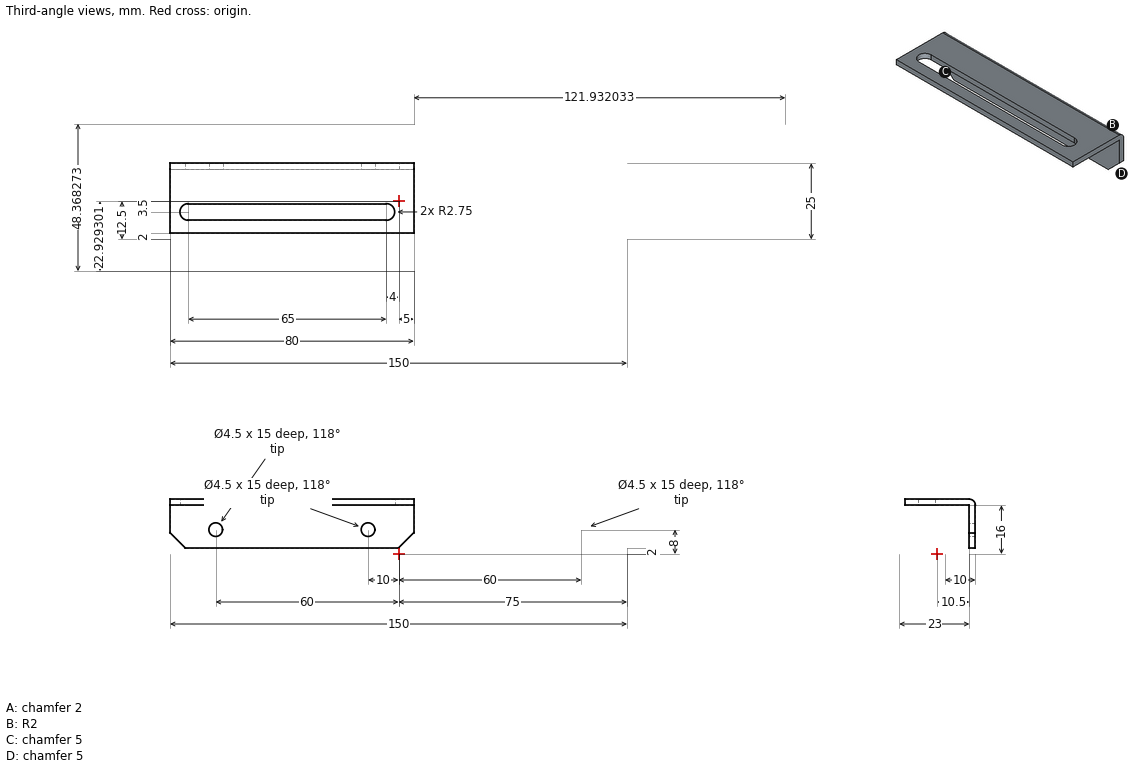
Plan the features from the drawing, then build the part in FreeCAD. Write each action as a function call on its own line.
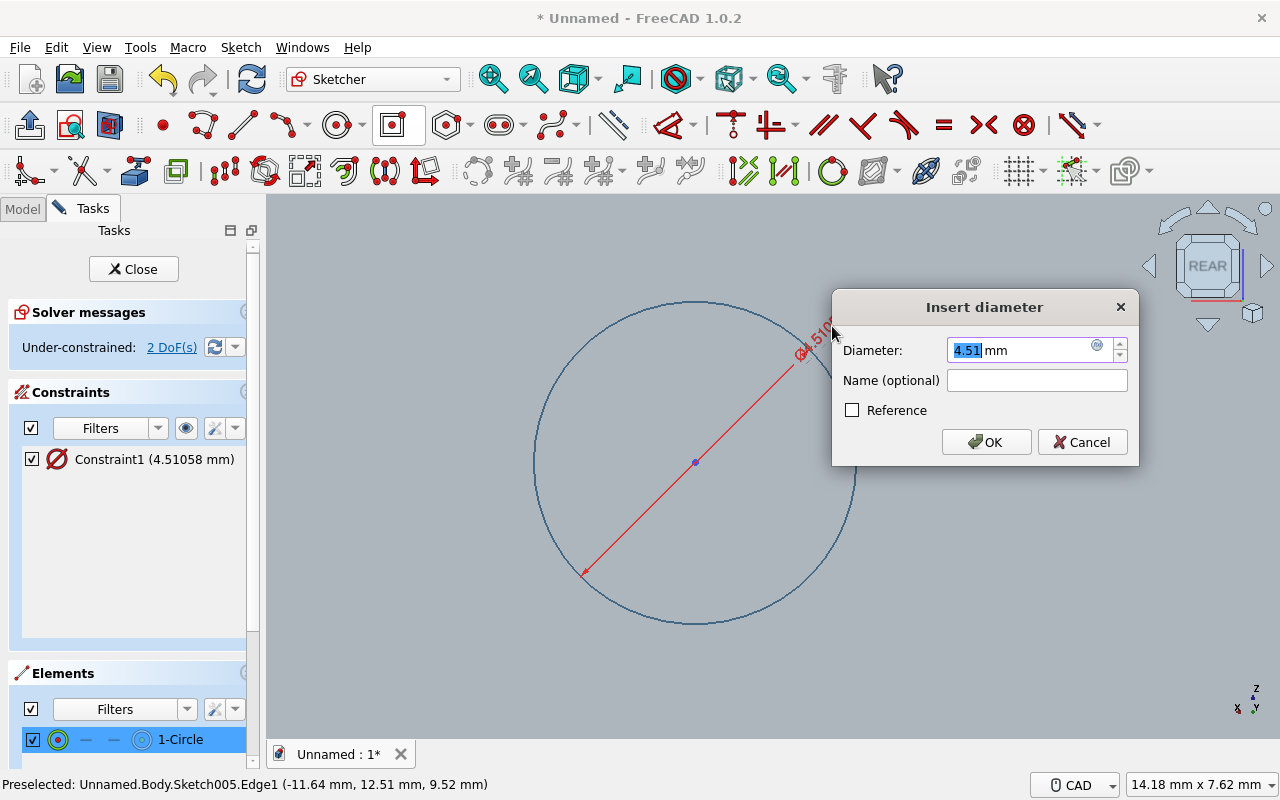
text(4.5)
key(Return)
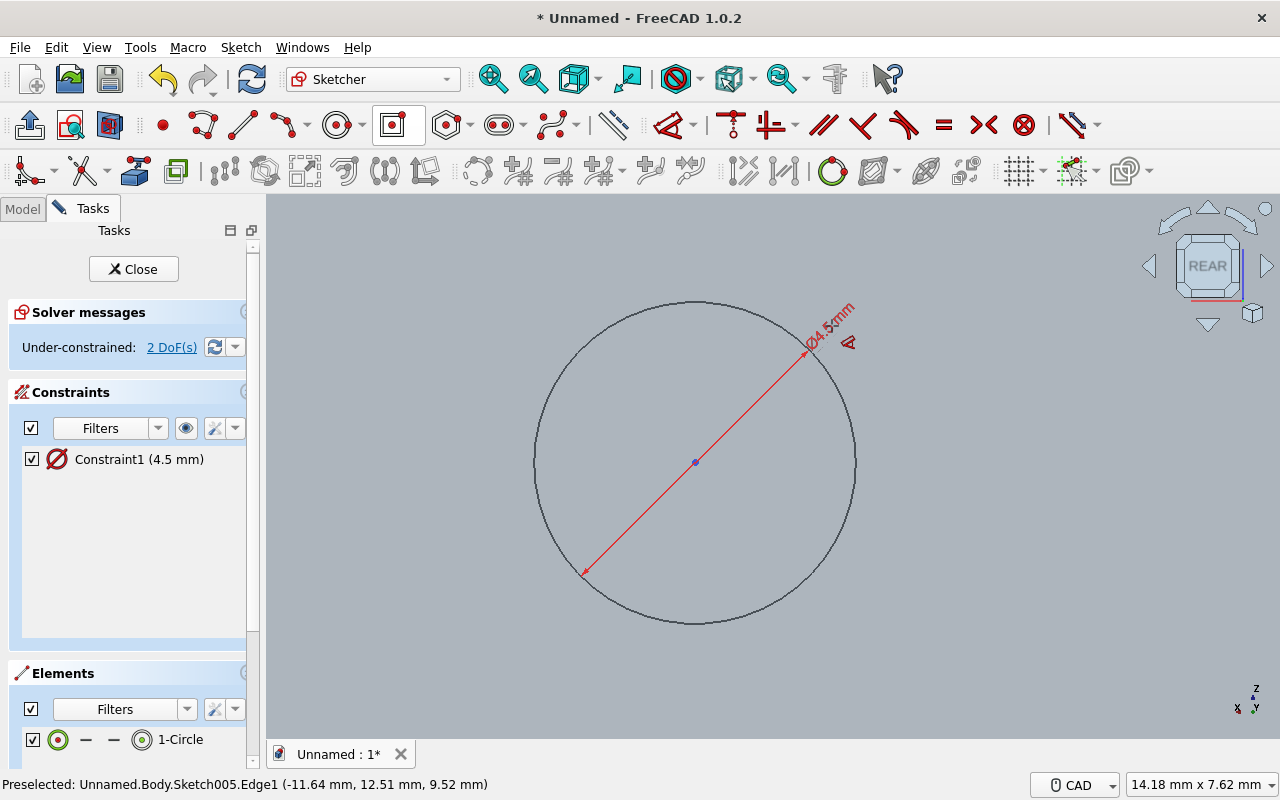
click(695, 463)
click(729, 587)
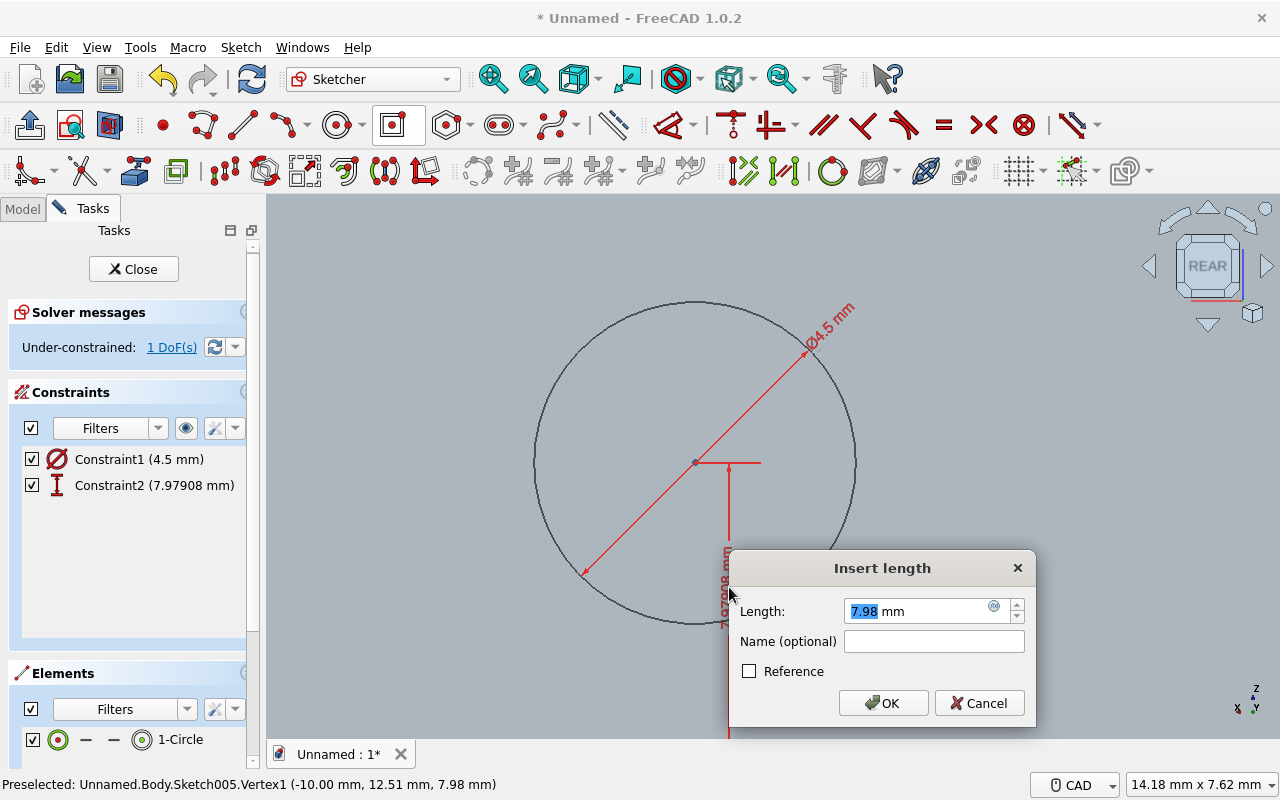
text(8)
key(Return)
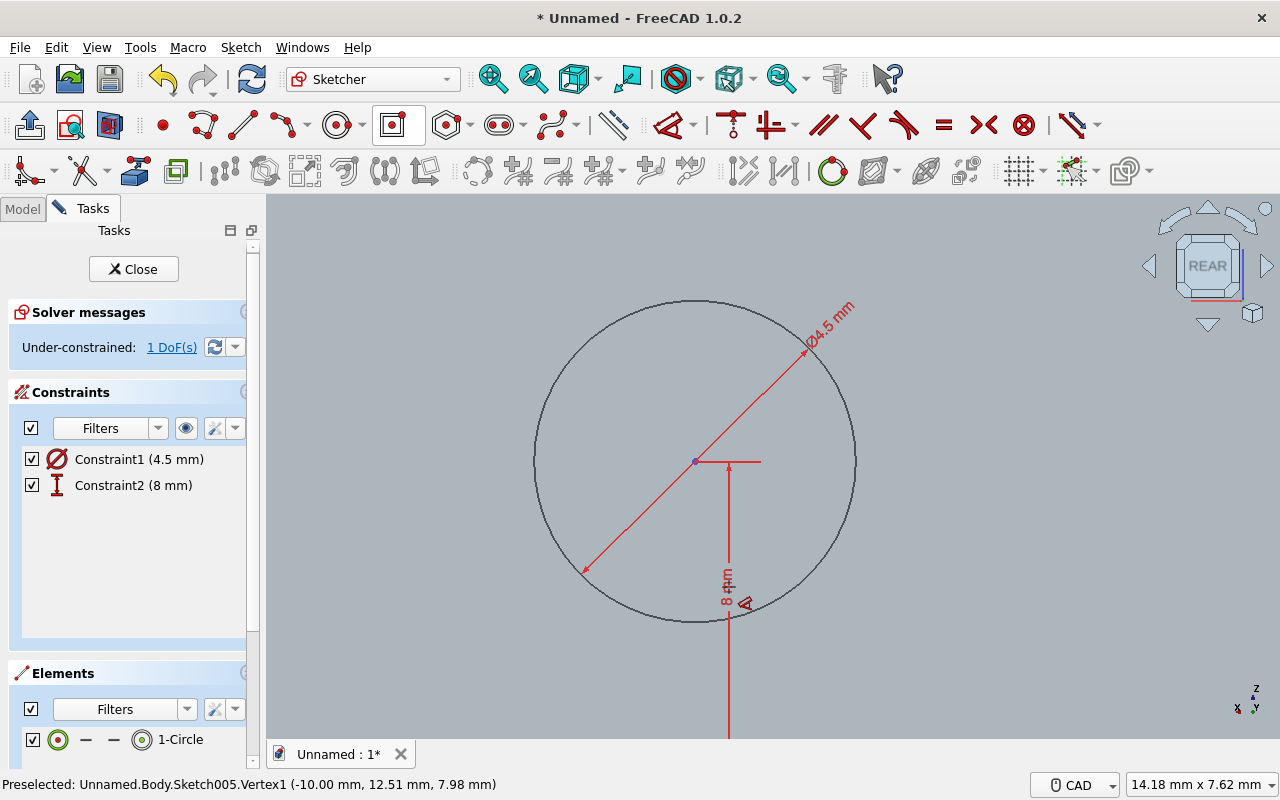
click(695, 462)
click(494, 428)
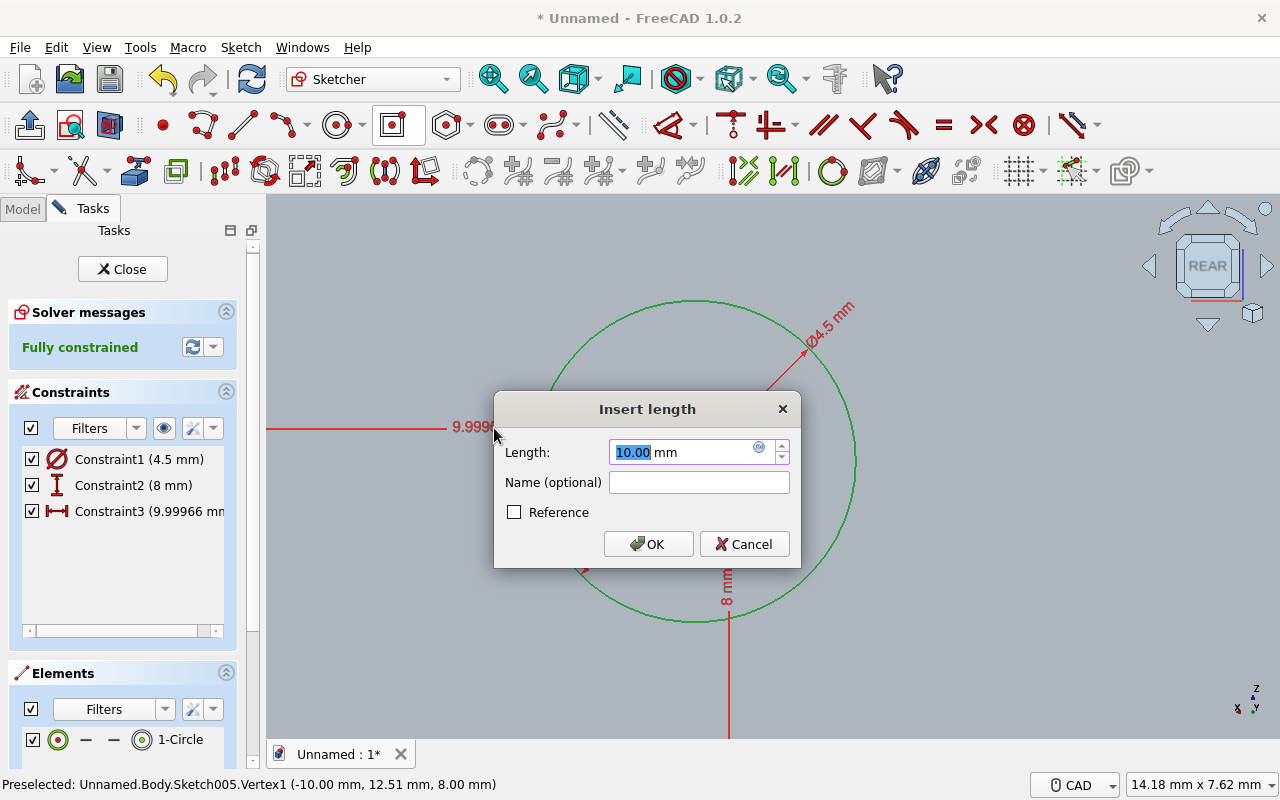
text(10)
key(Return)
key(Escape)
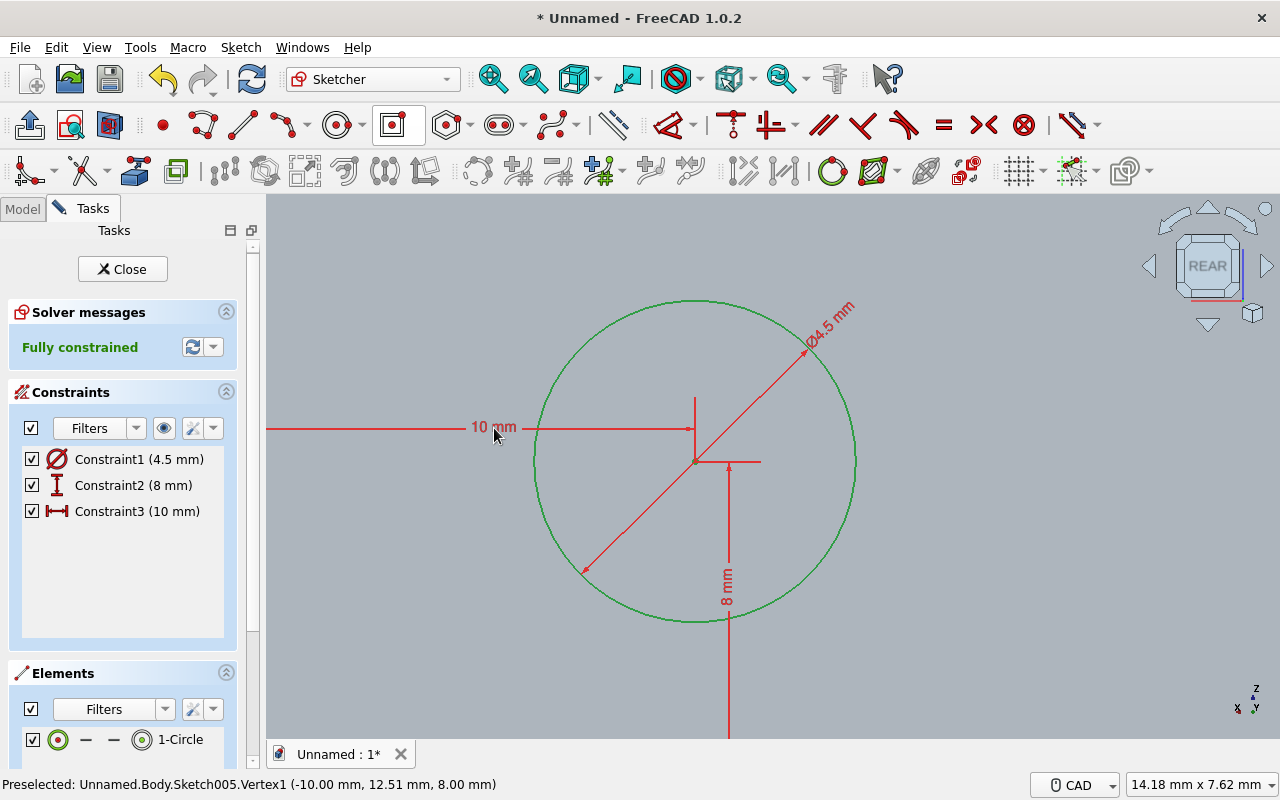
click(123, 269)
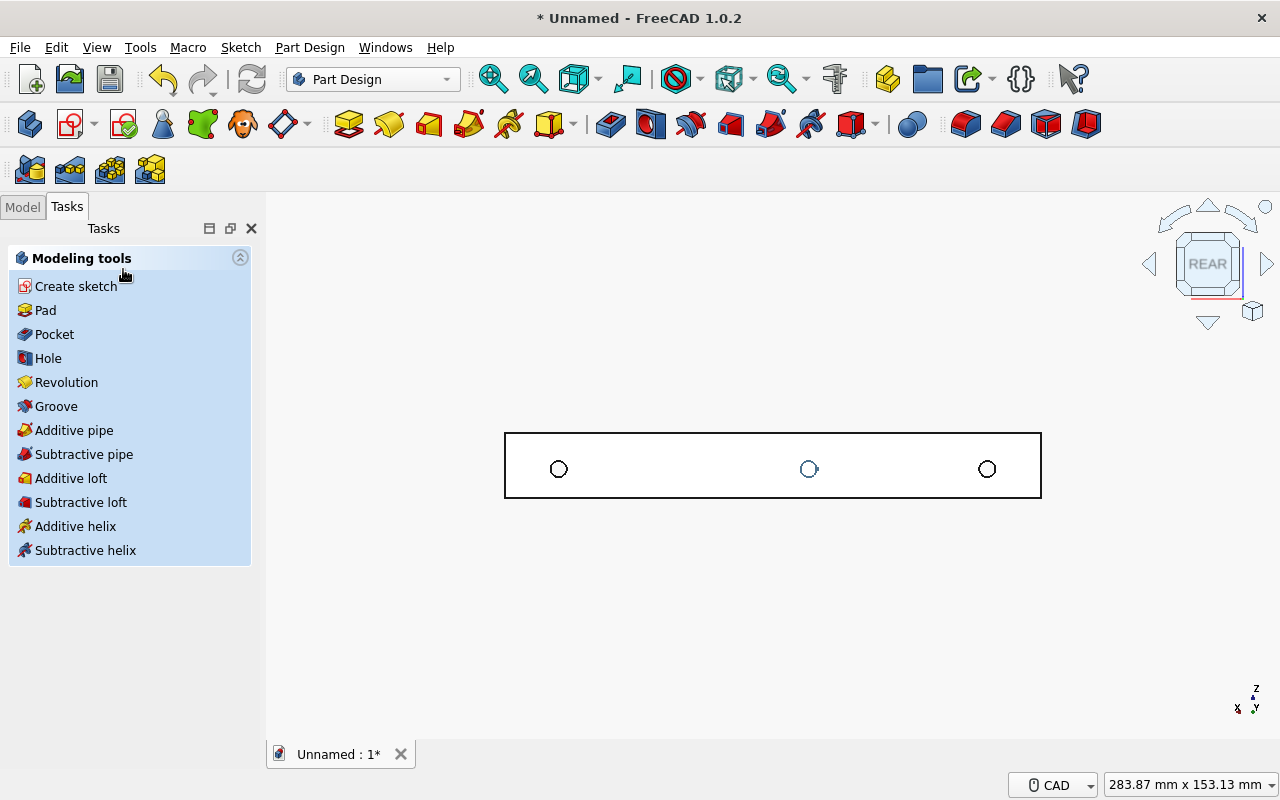
click(652, 124)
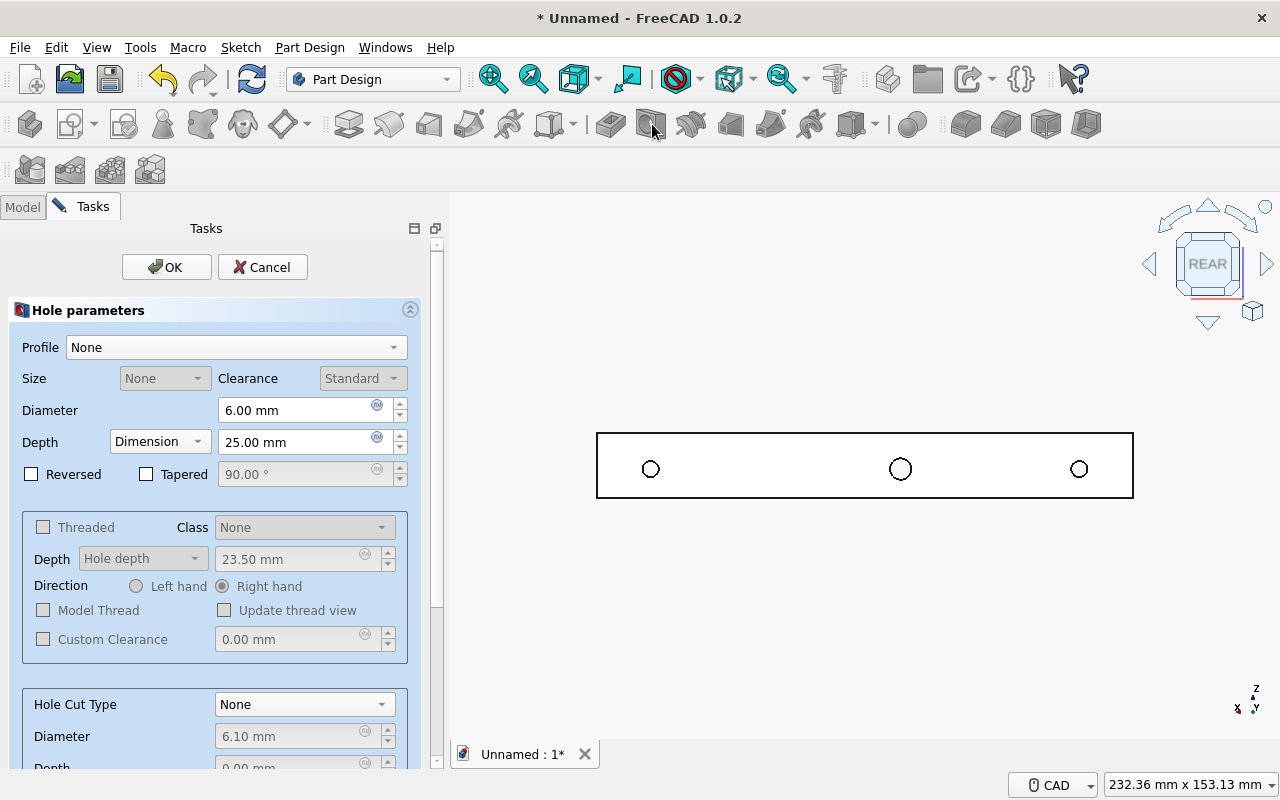
triple_click(305, 410)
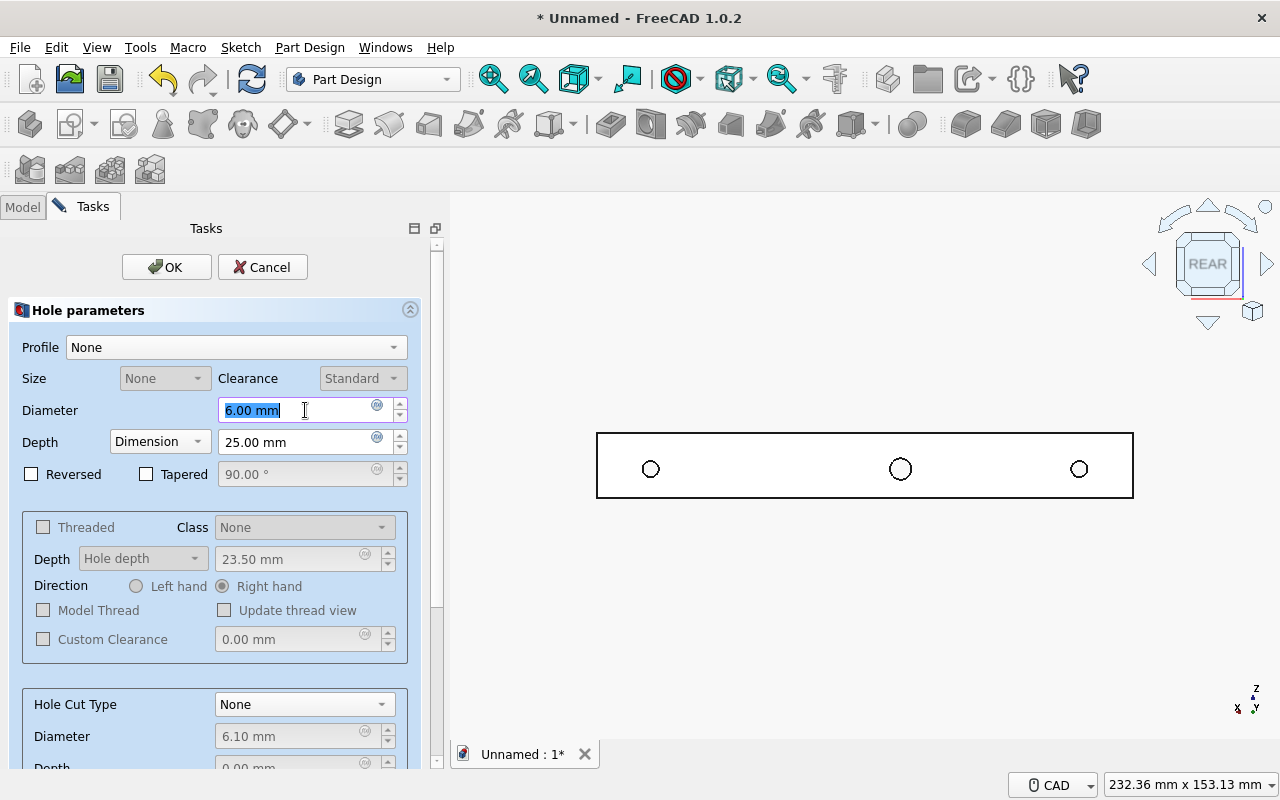
text(4.5)
key(Tab)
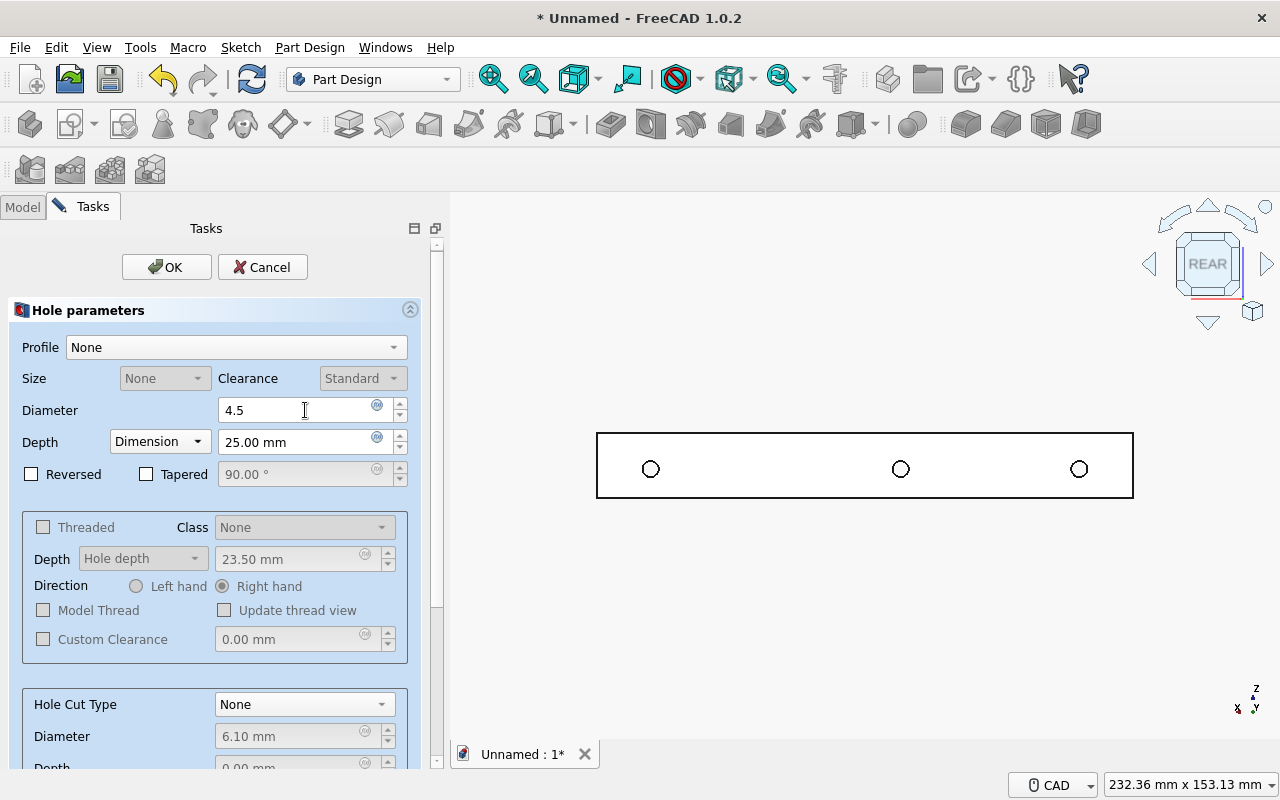
triple_click(305, 442)